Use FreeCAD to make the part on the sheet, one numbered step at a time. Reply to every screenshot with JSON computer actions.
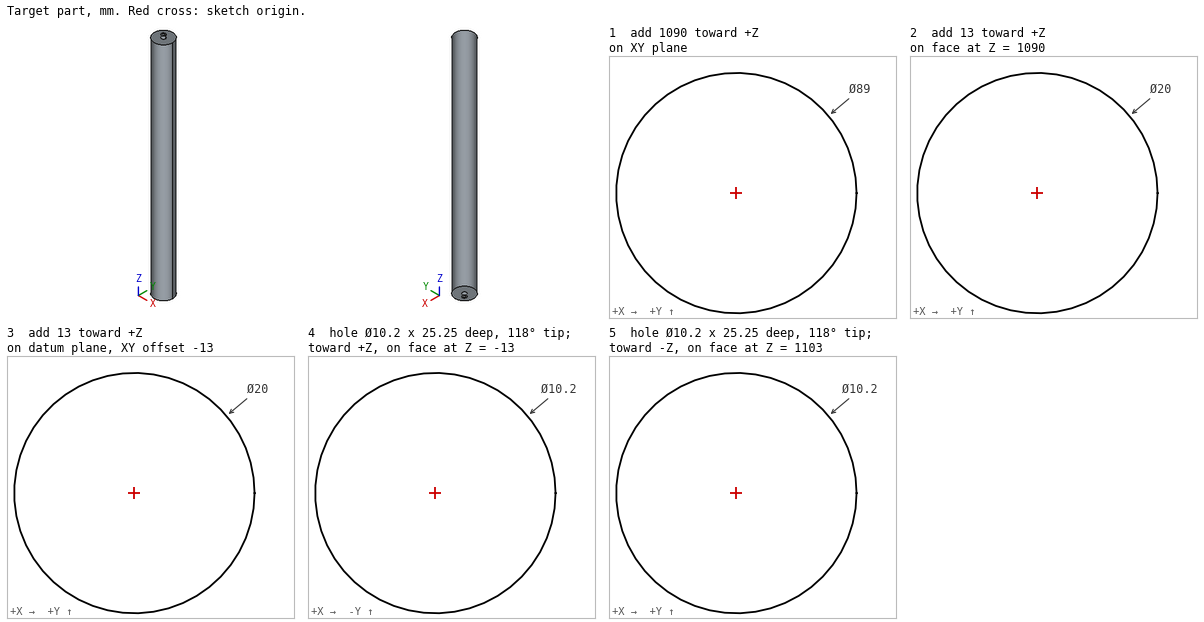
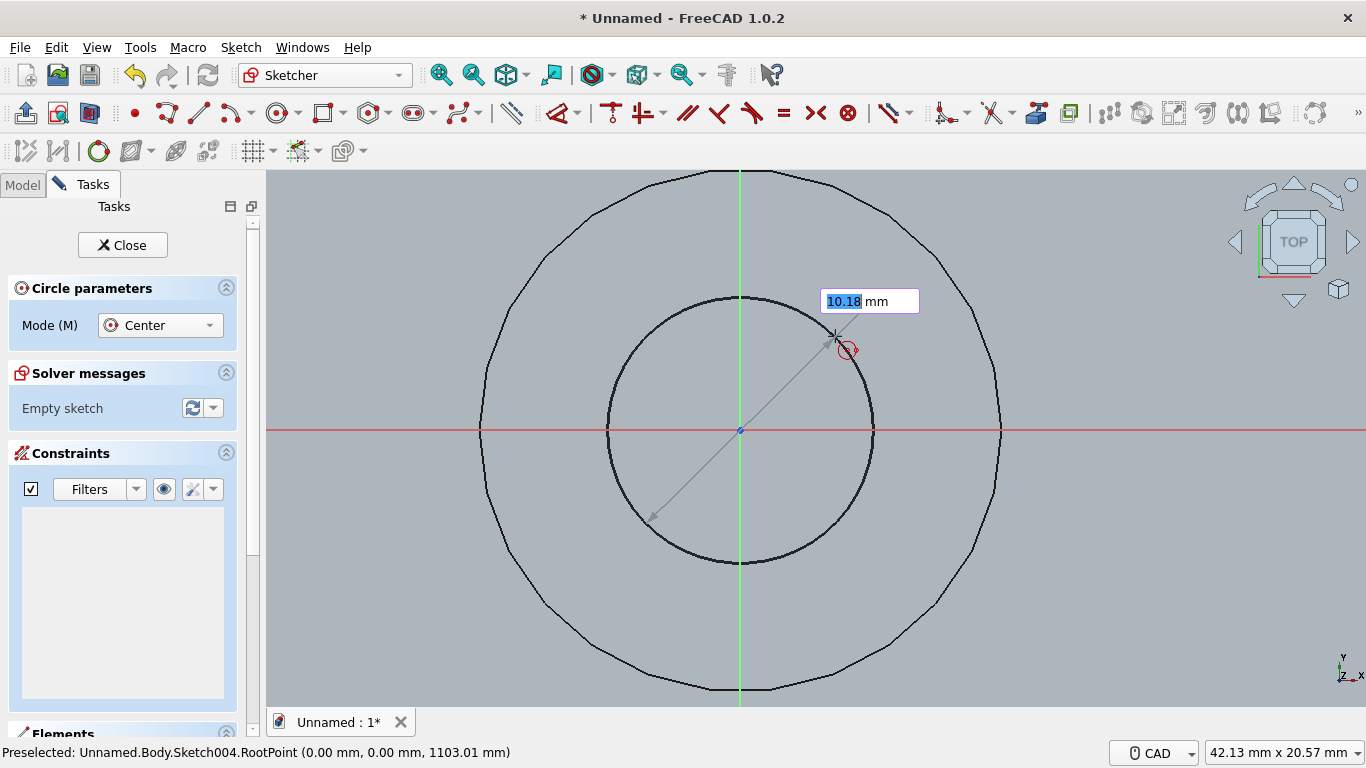
{"action": "type", "text": "10.2"}
{"action": "key", "text": "Return"}
{"action": "key", "text": "Escape"}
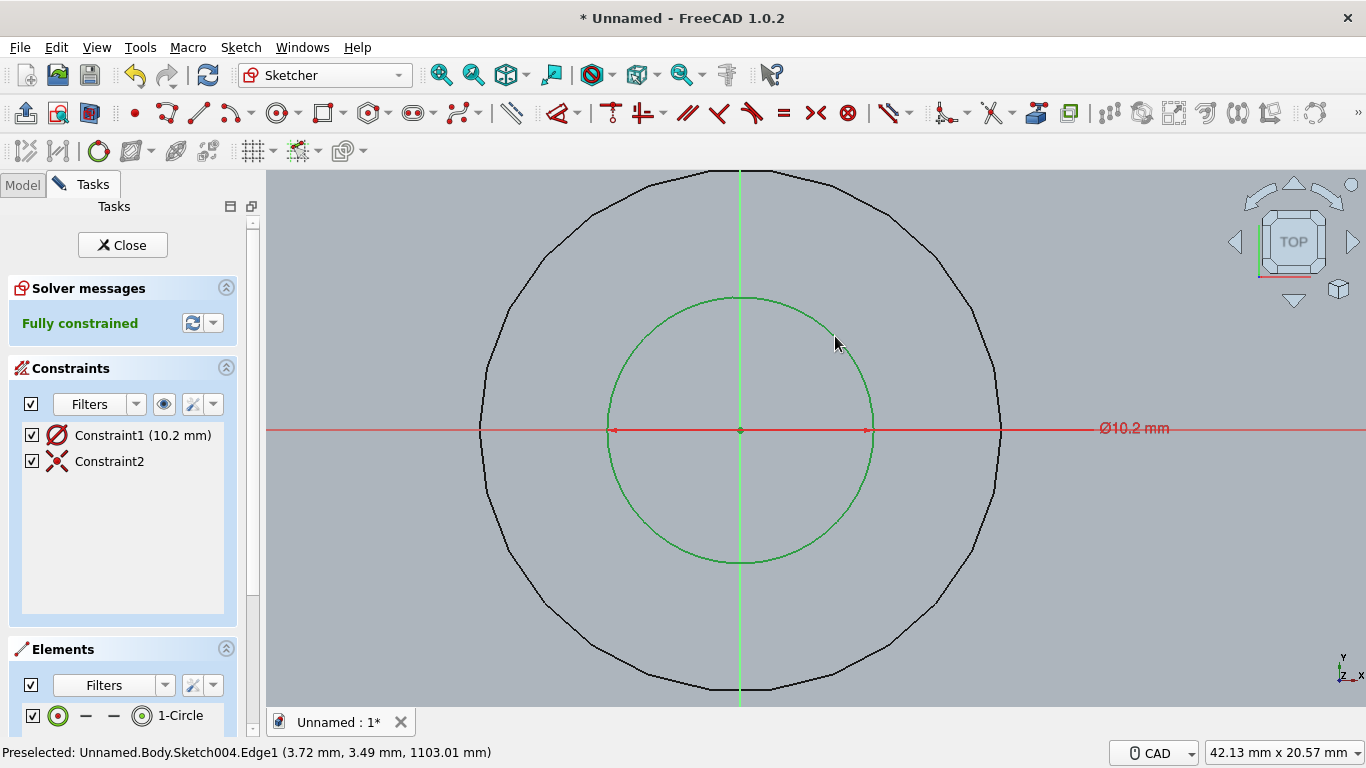
{"action": "left_click", "coordinate": [123, 245]}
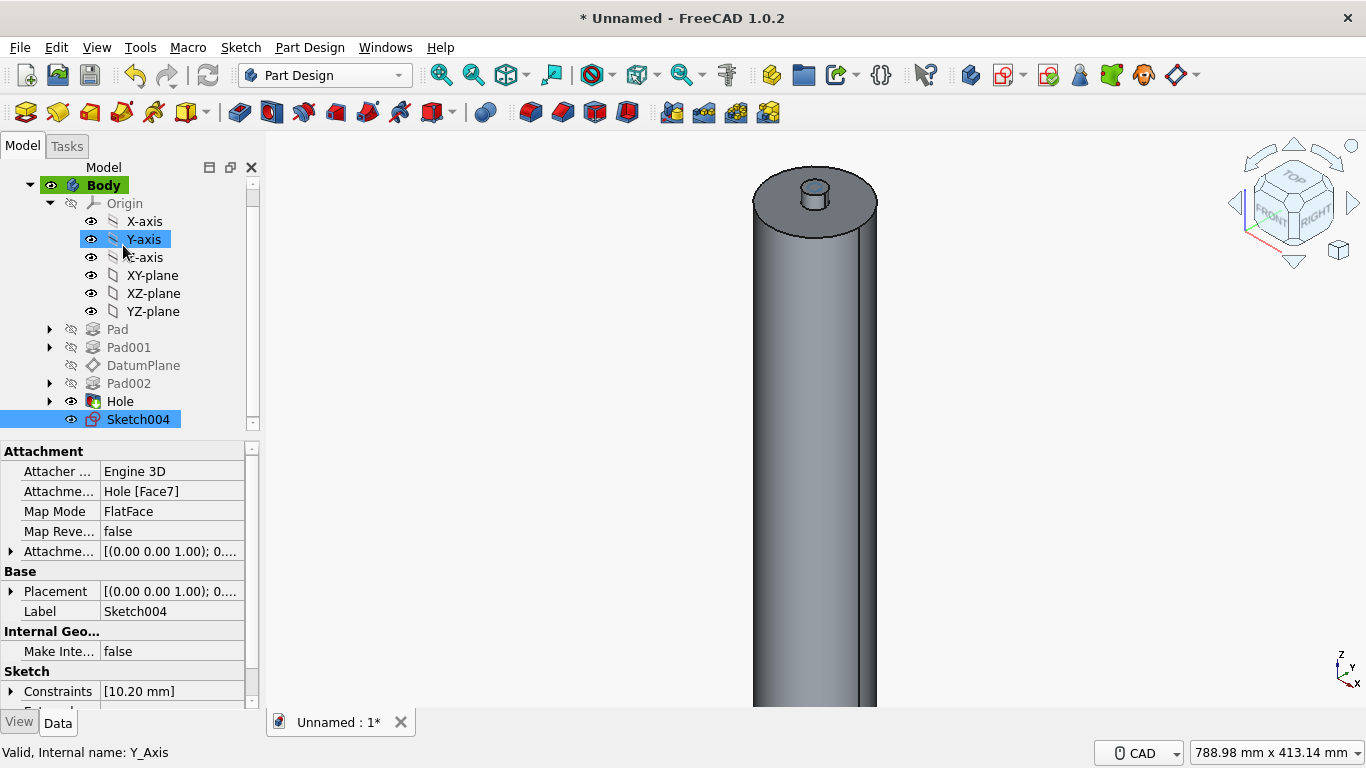
{"action": "left_click", "coordinate": [272, 112]}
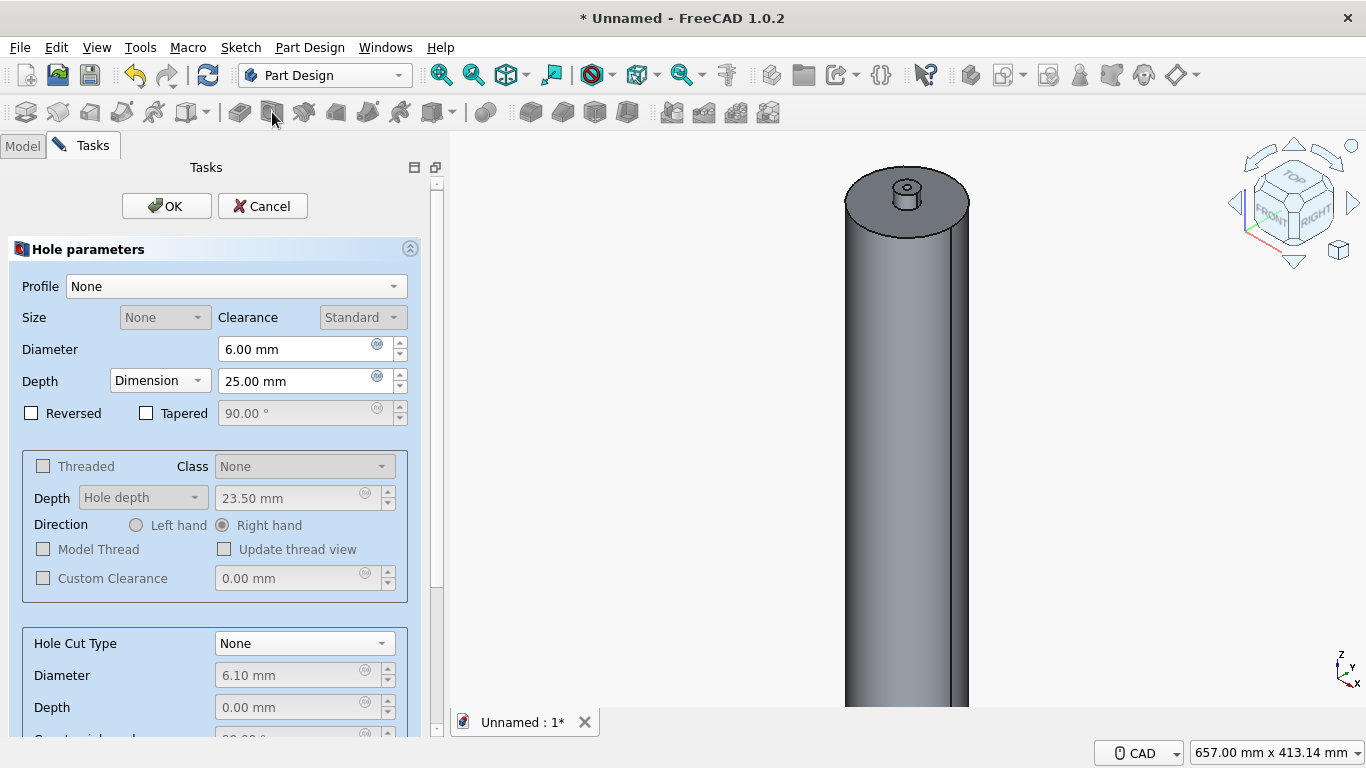
{"action": "triple_click", "coordinate": [305, 349]}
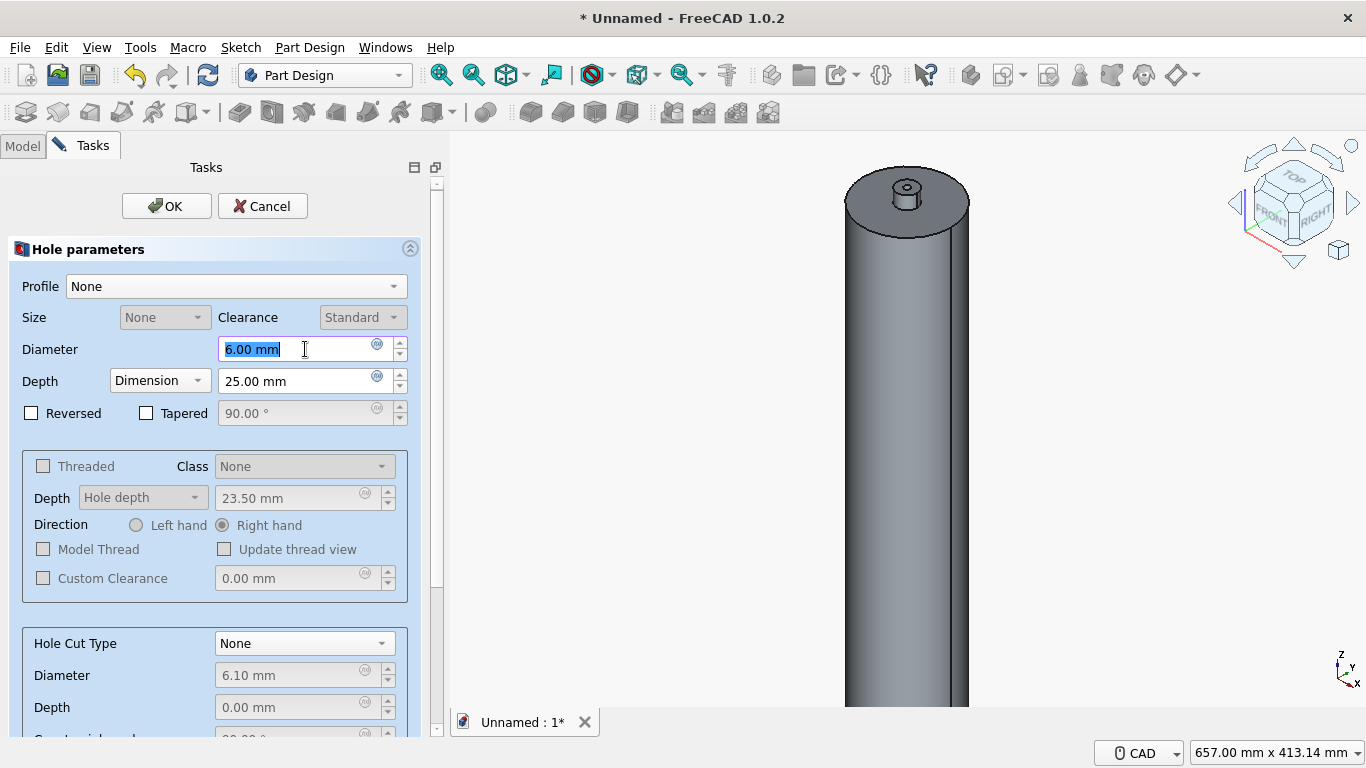
{"action": "type", "text": "10.2"}
{"action": "key", "text": "Tab"}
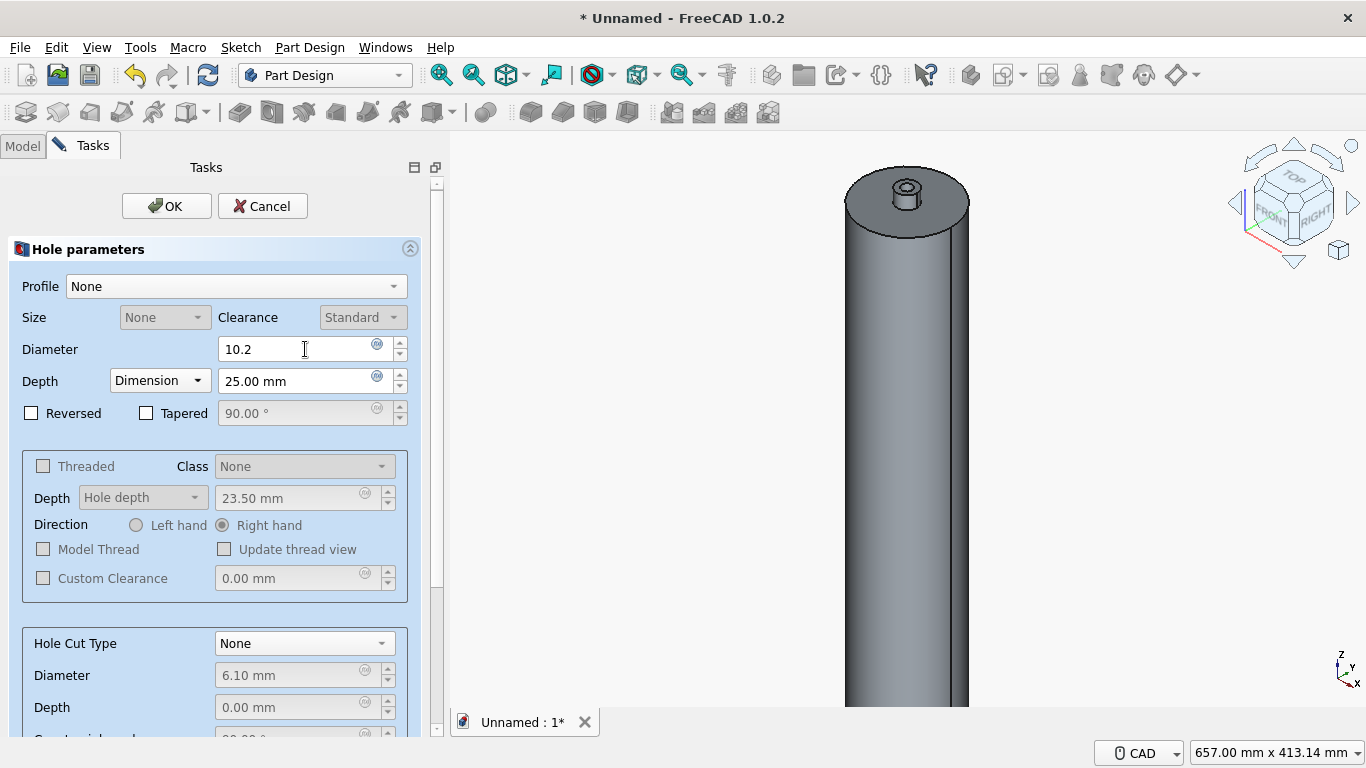
{"action": "triple_click", "coordinate": [305, 381]}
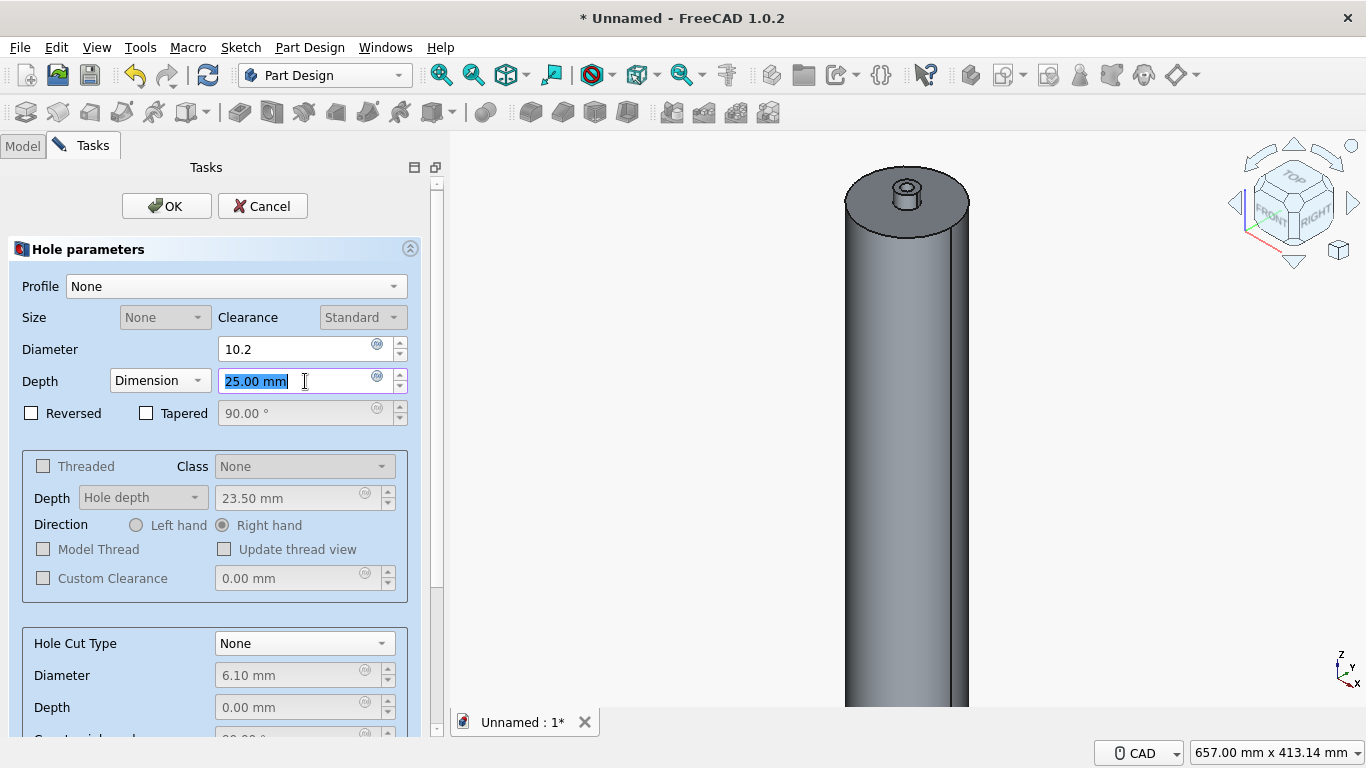
{"action": "type", "text": "25.25"}
{"action": "key", "text": "Tab"}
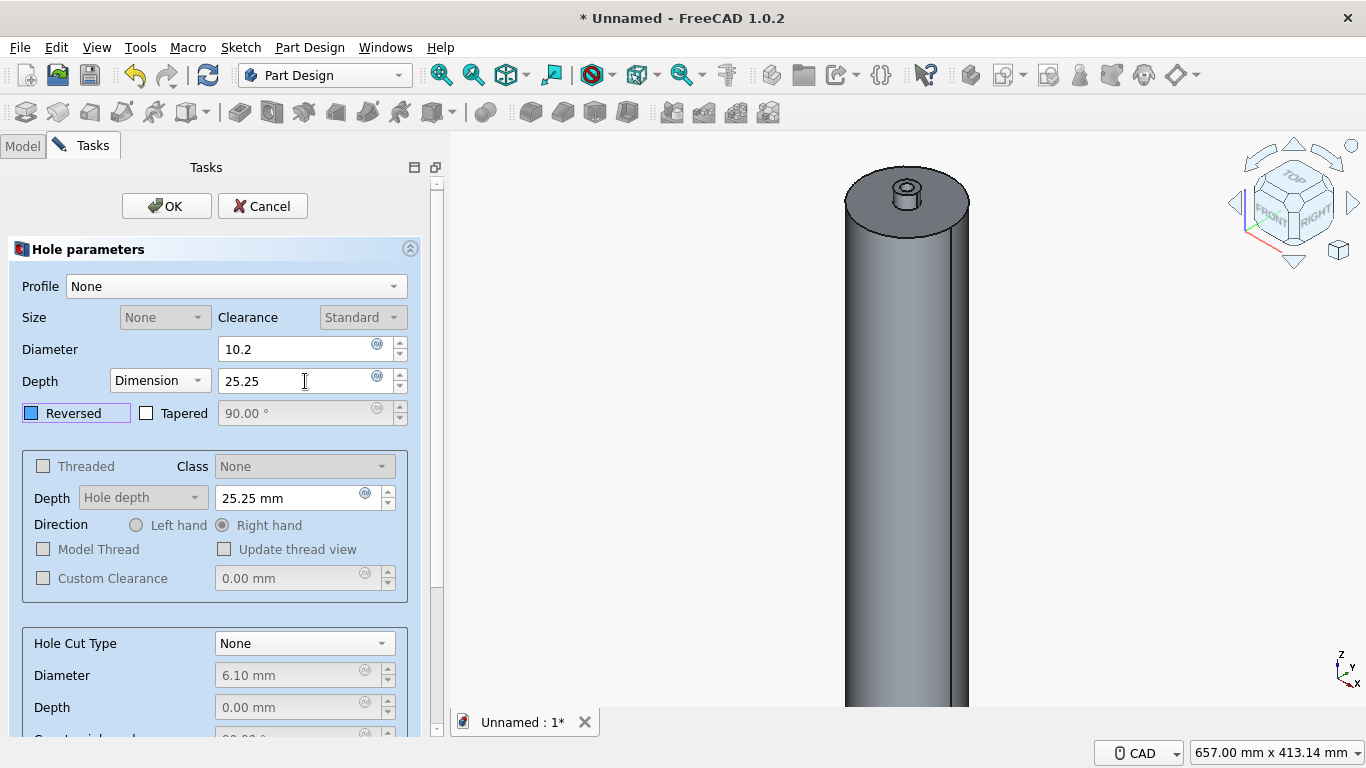
{"action": "left_click", "coordinate": [167, 206]}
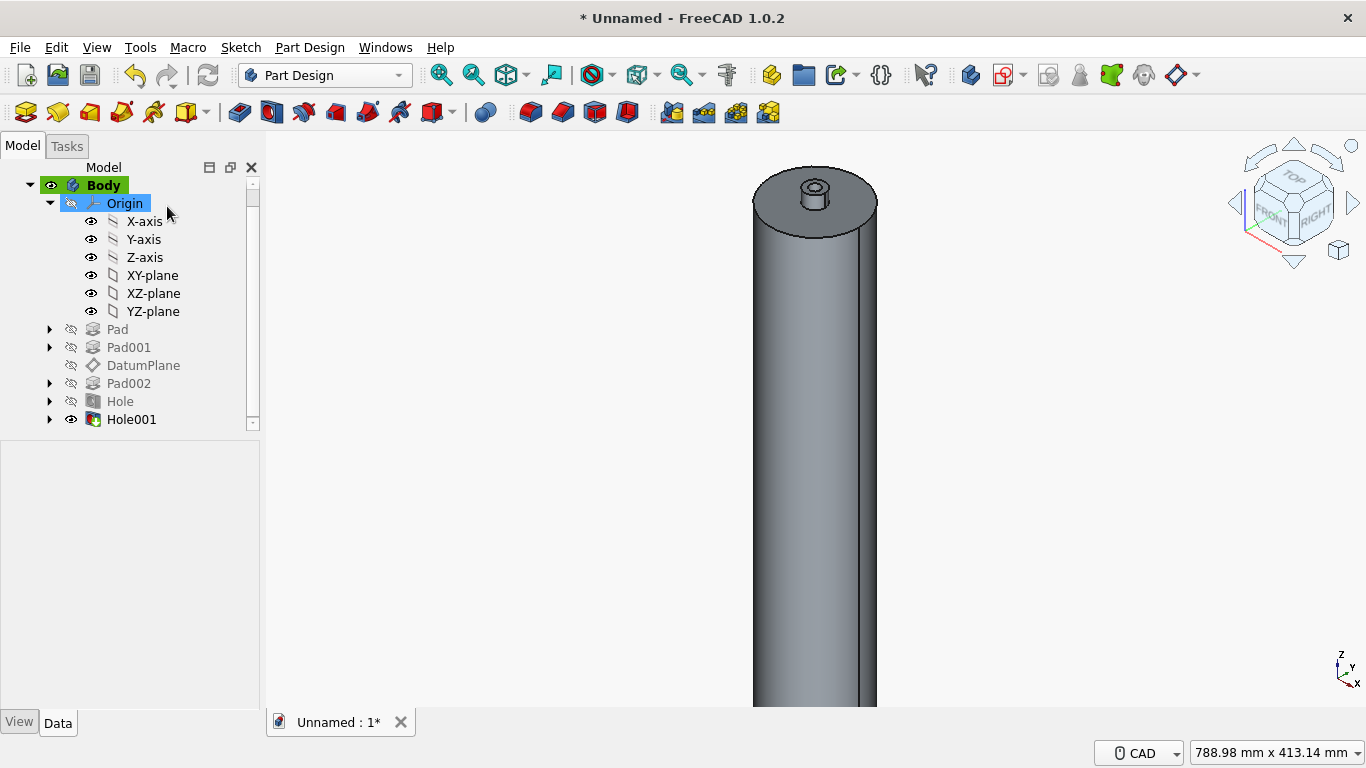
{"action": "key", "text": "v f"}